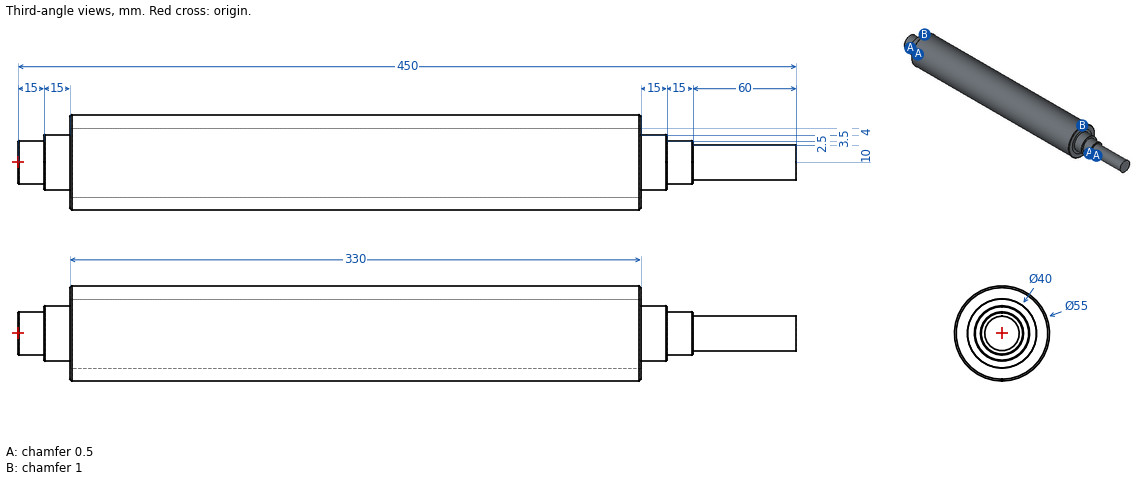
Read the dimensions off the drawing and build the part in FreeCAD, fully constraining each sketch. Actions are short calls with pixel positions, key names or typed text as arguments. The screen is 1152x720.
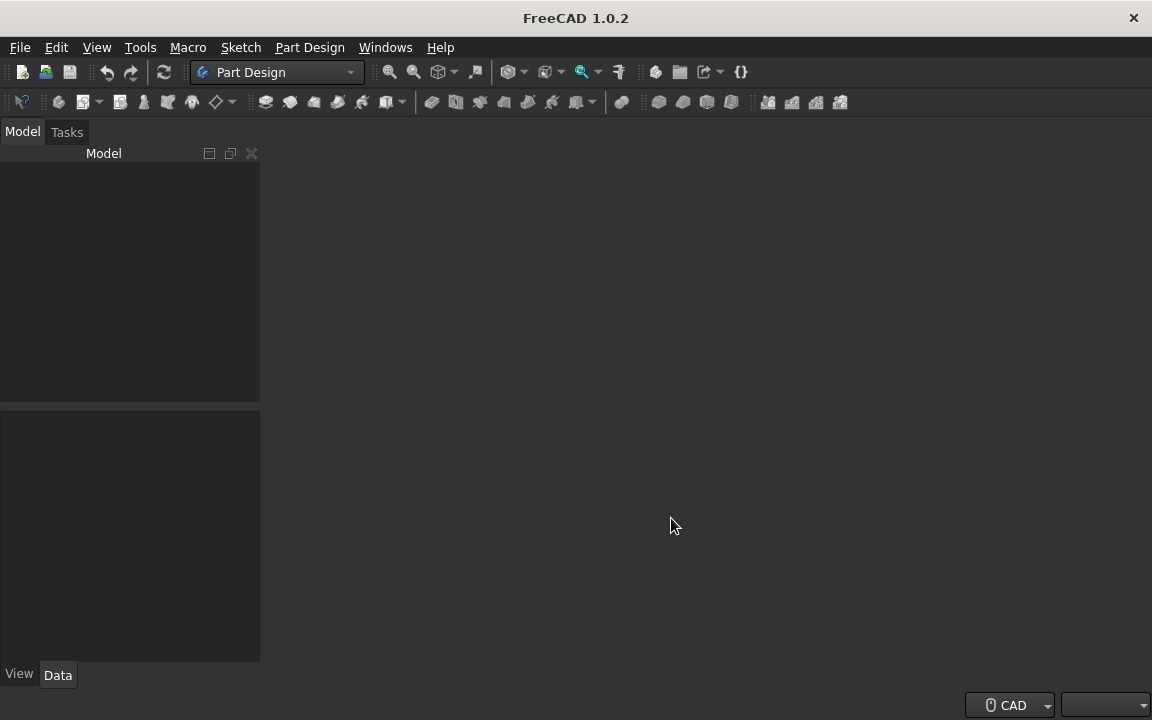
click(22, 72)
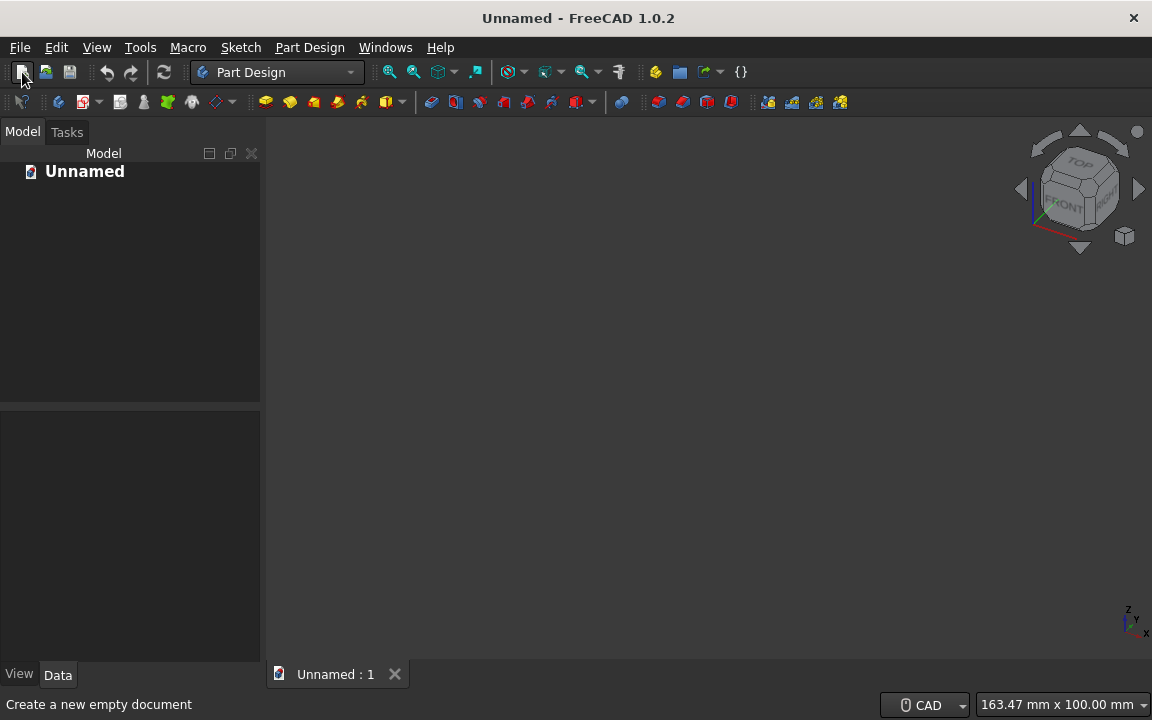
click(84, 102)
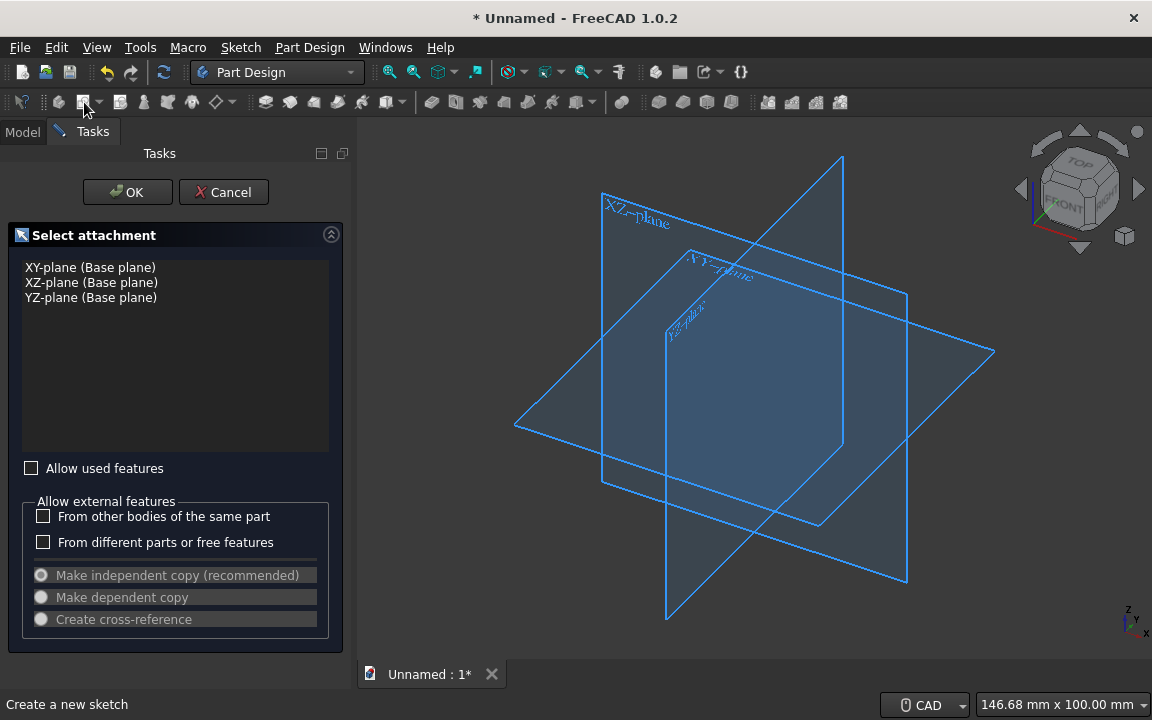
click(82, 268)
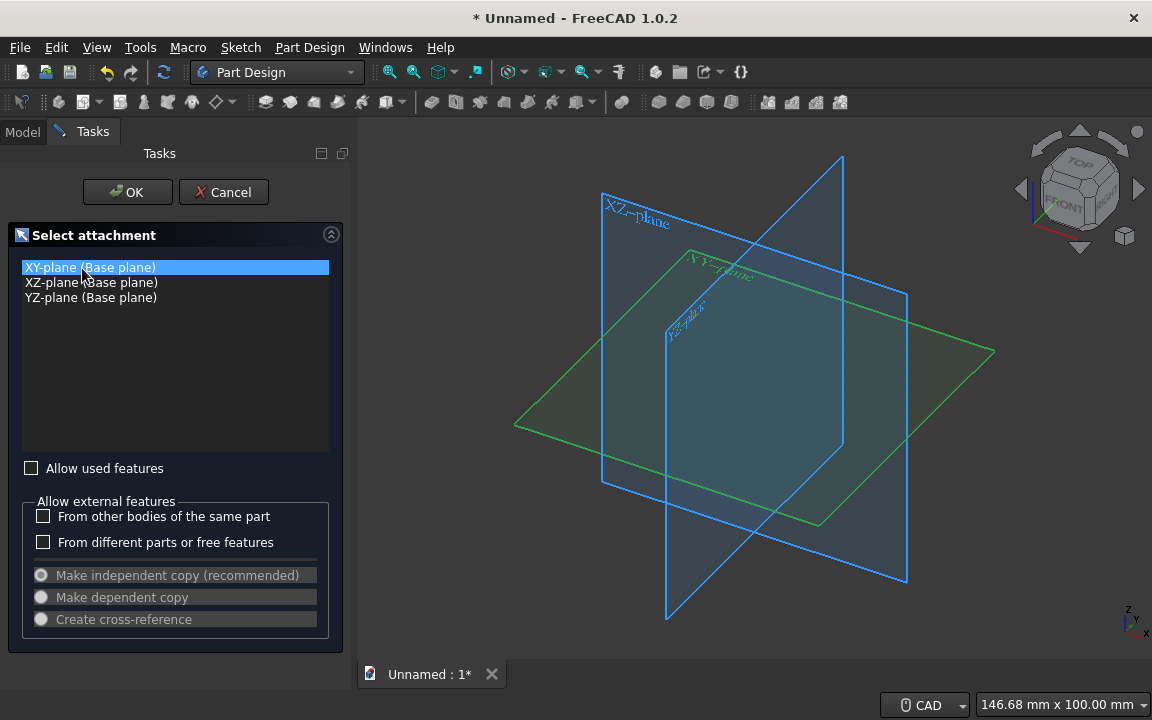
click(128, 192)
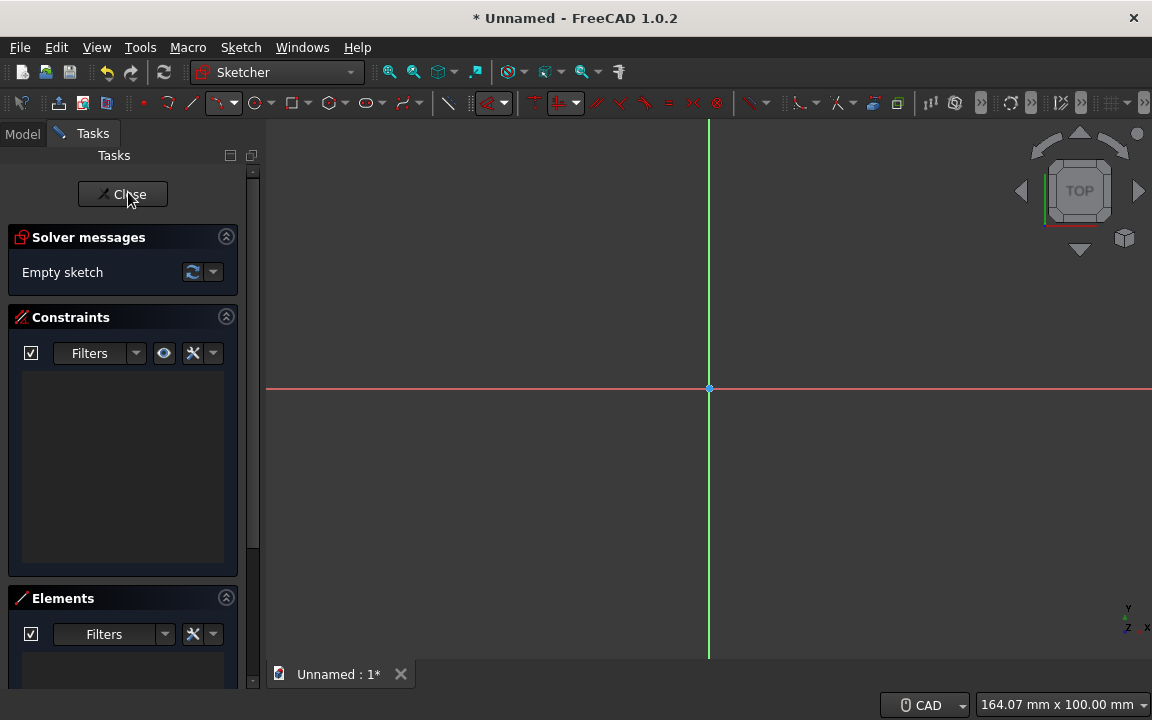
scroll(316, 403, down, 8)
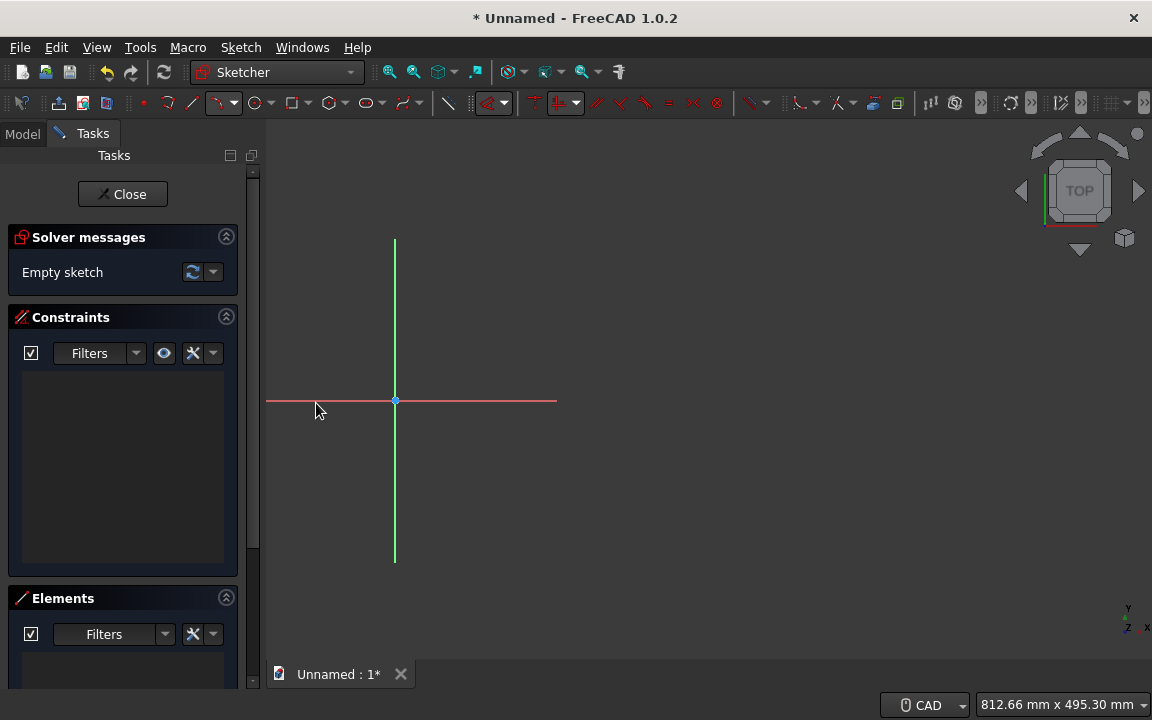
click(168, 104)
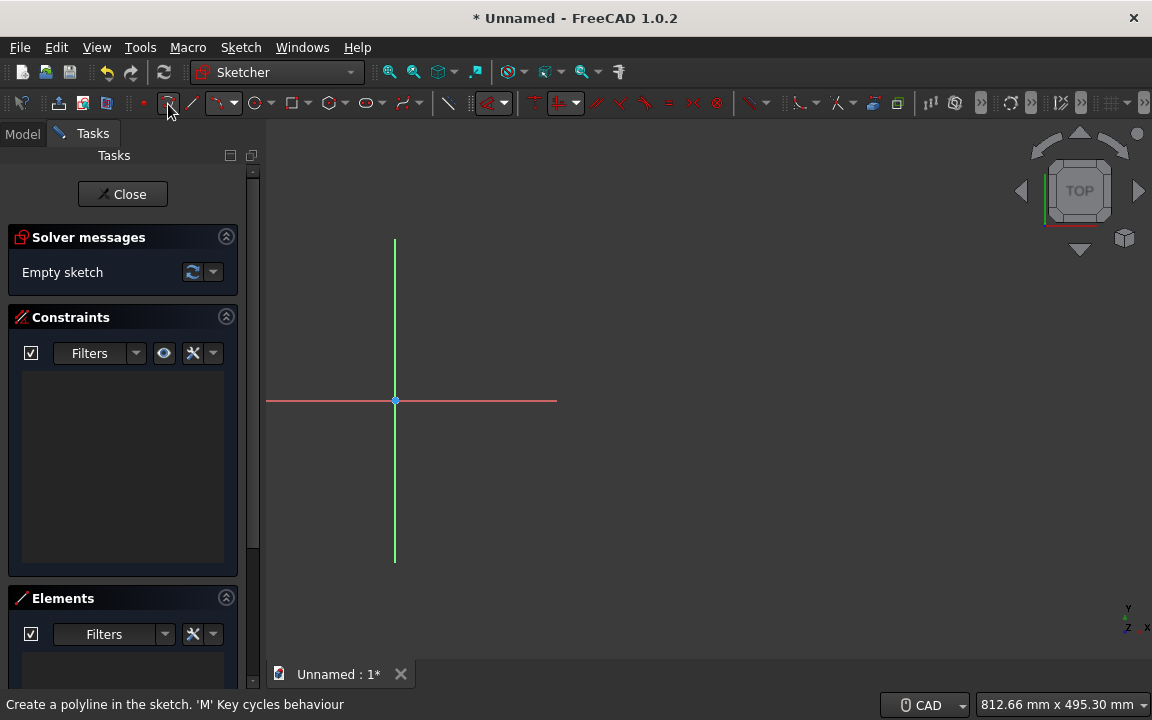
click(395, 401)
click(886, 392)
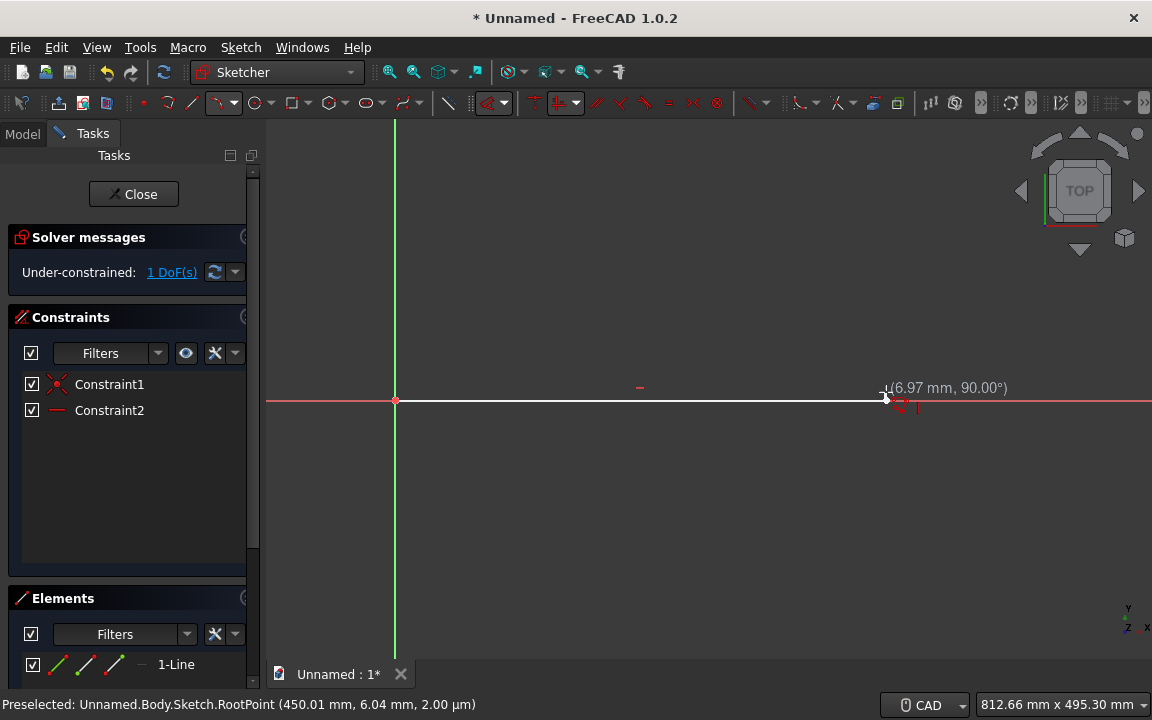
scroll(886, 390, up, 2)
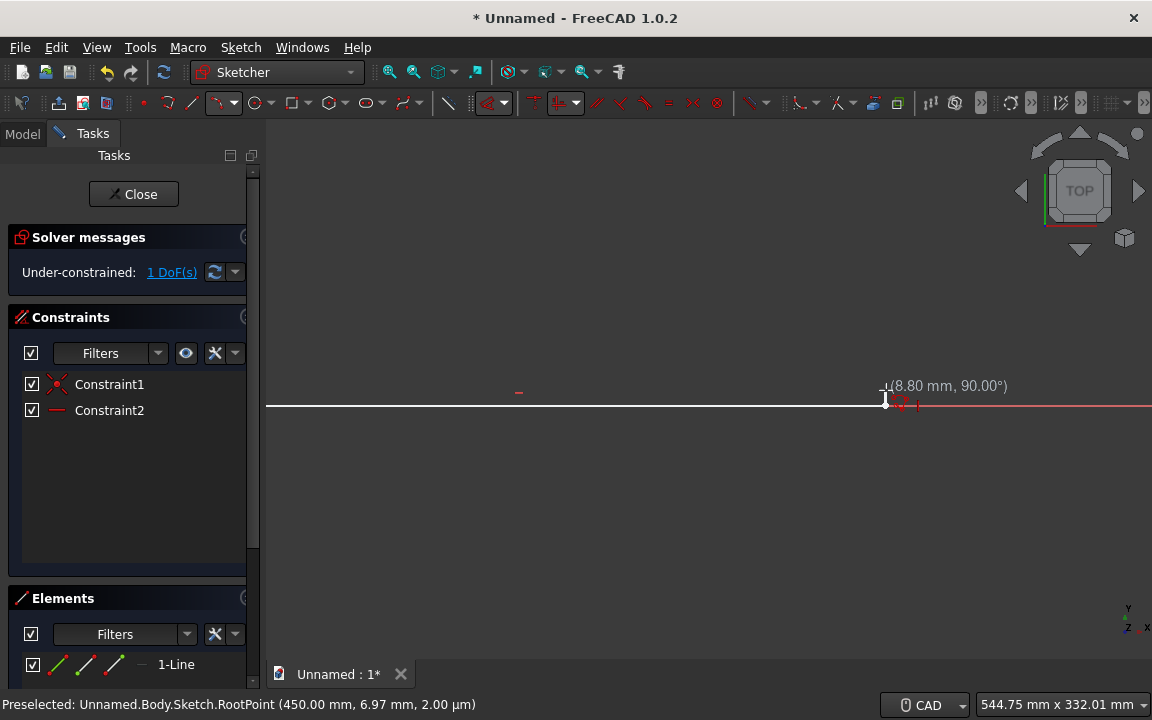
click(886, 389)
click(788, 389)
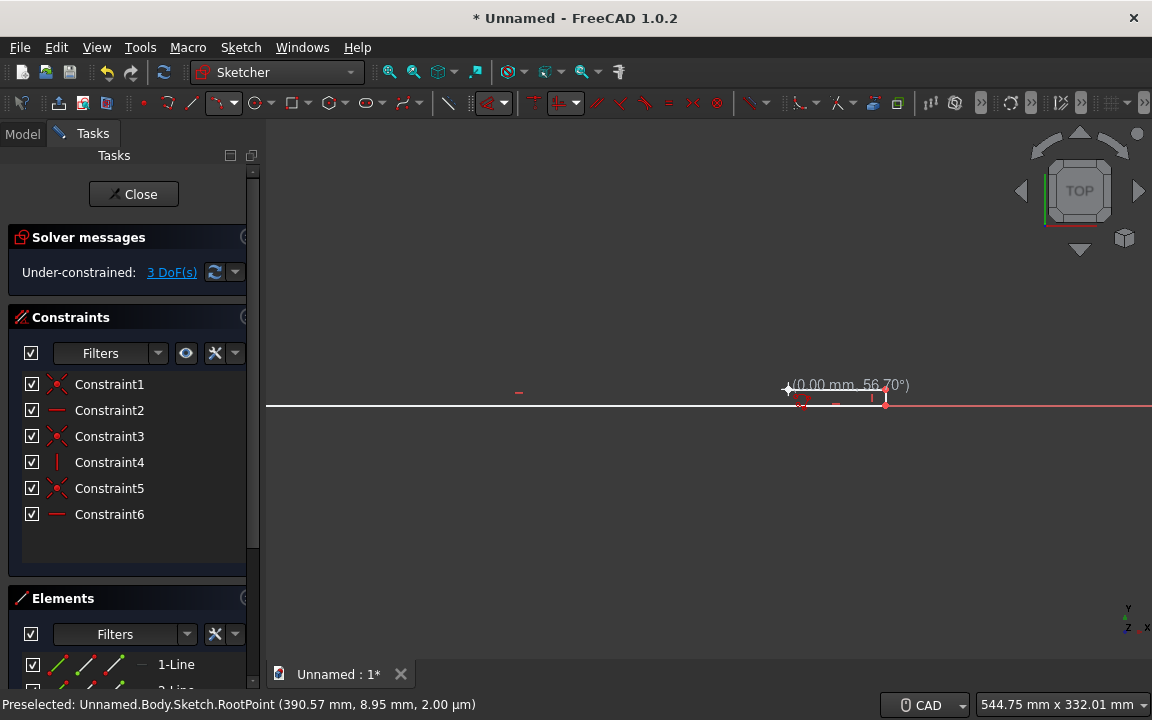
scroll(788, 385, up, 7)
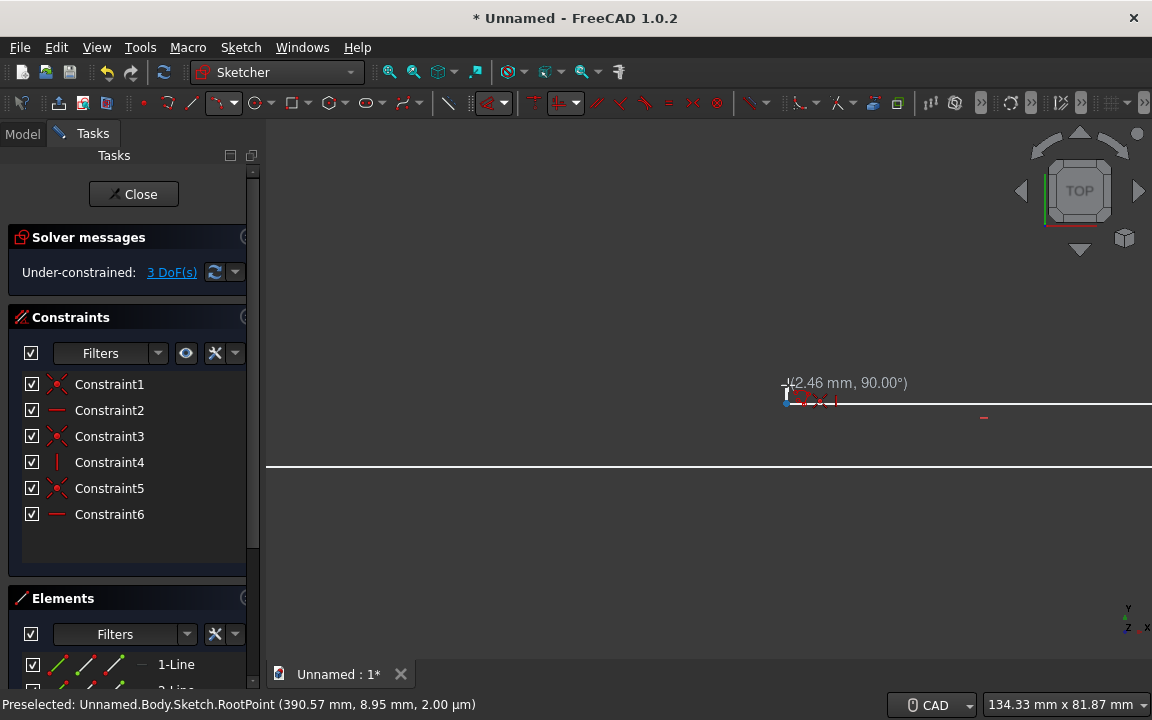
click(786, 384)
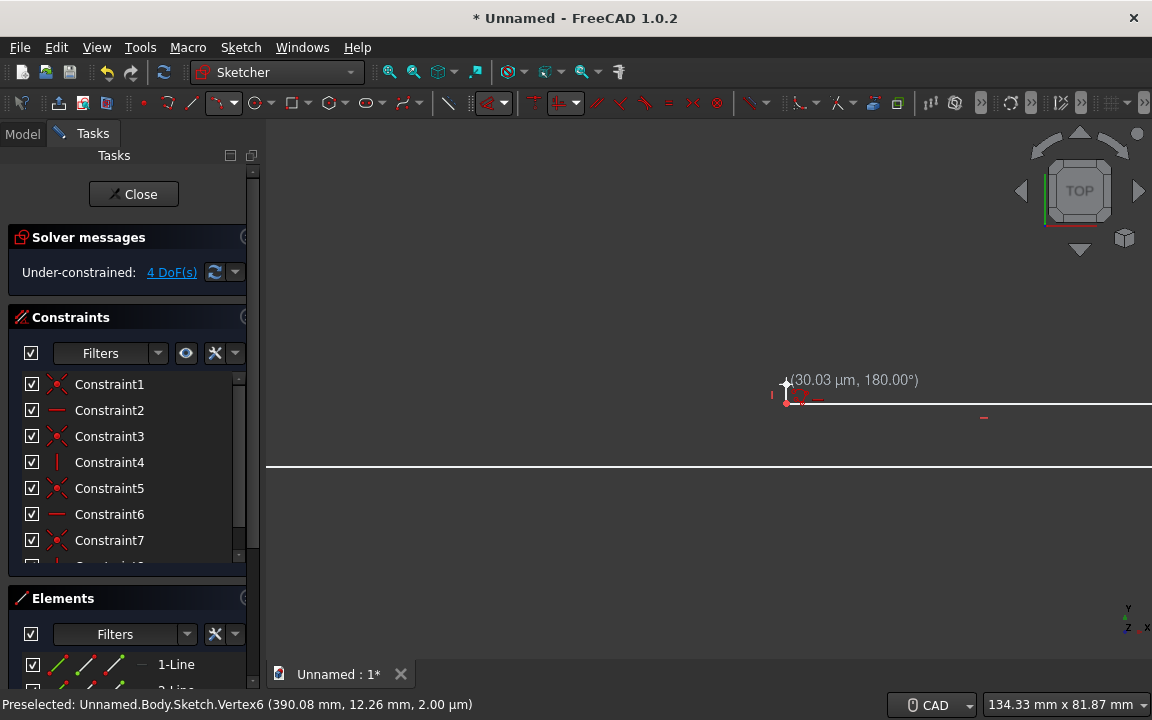
scroll(827, 387, down, 9)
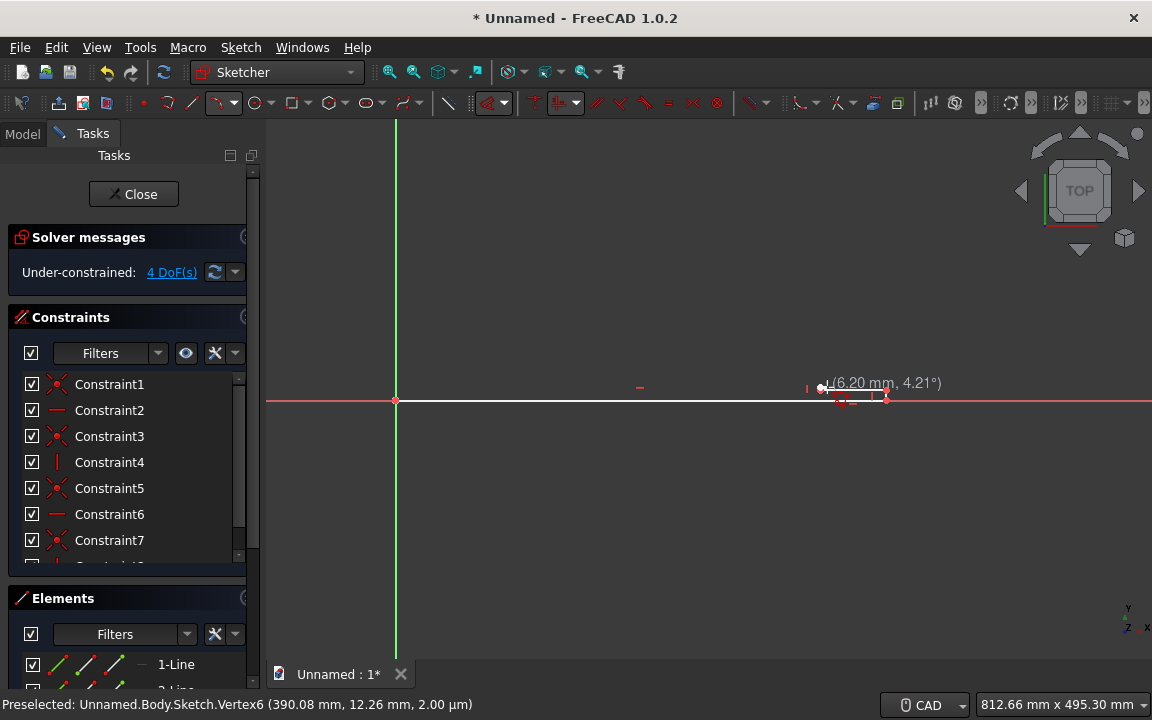
click(804, 387)